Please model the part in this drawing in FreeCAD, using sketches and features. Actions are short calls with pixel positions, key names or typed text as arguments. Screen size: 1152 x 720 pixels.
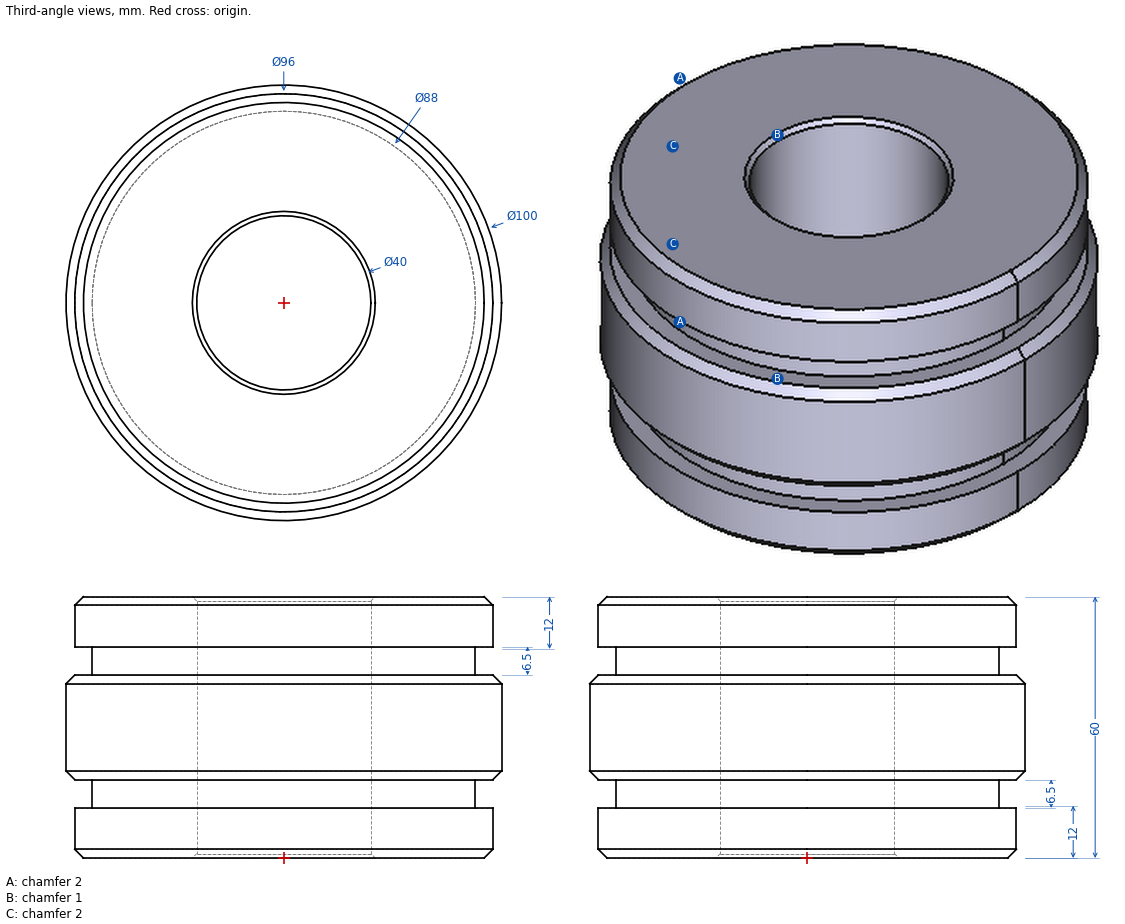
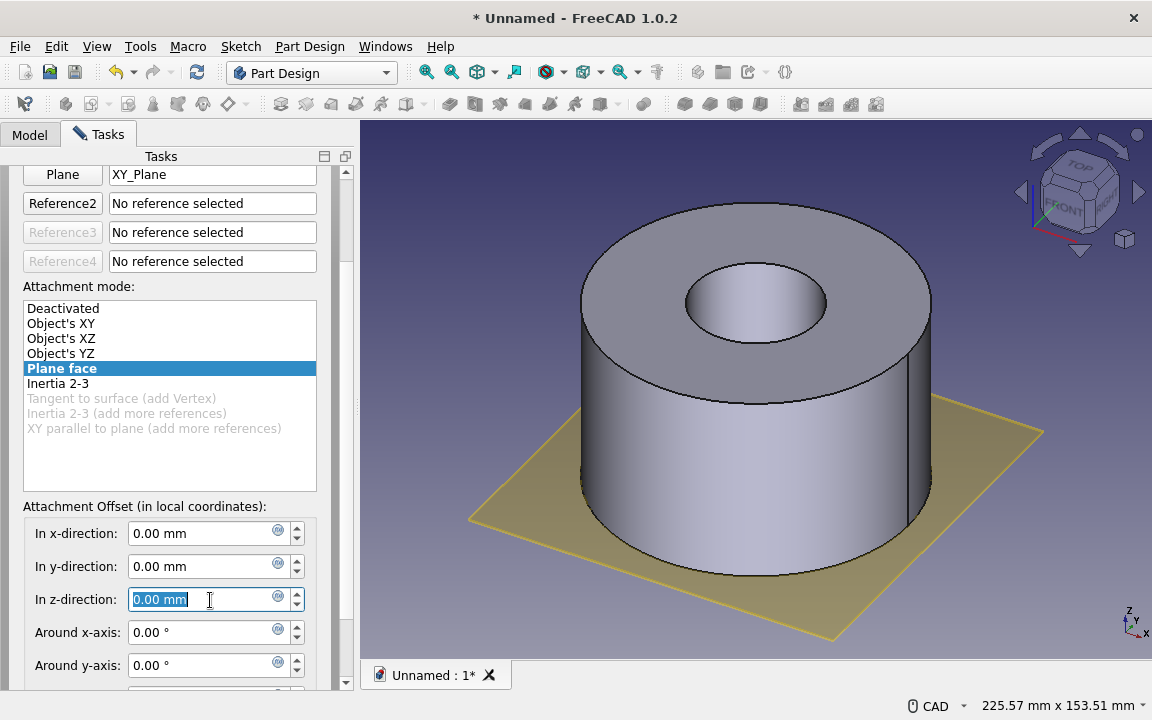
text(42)
key(Tab)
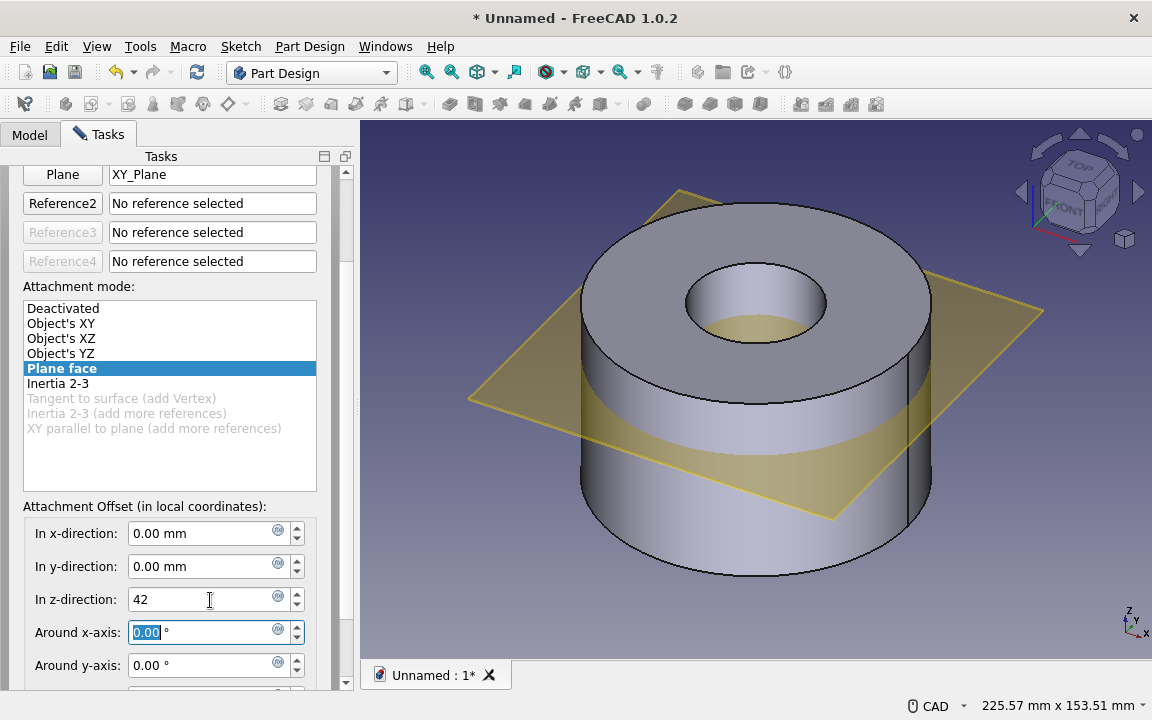
scroll(346, 428, up, 3)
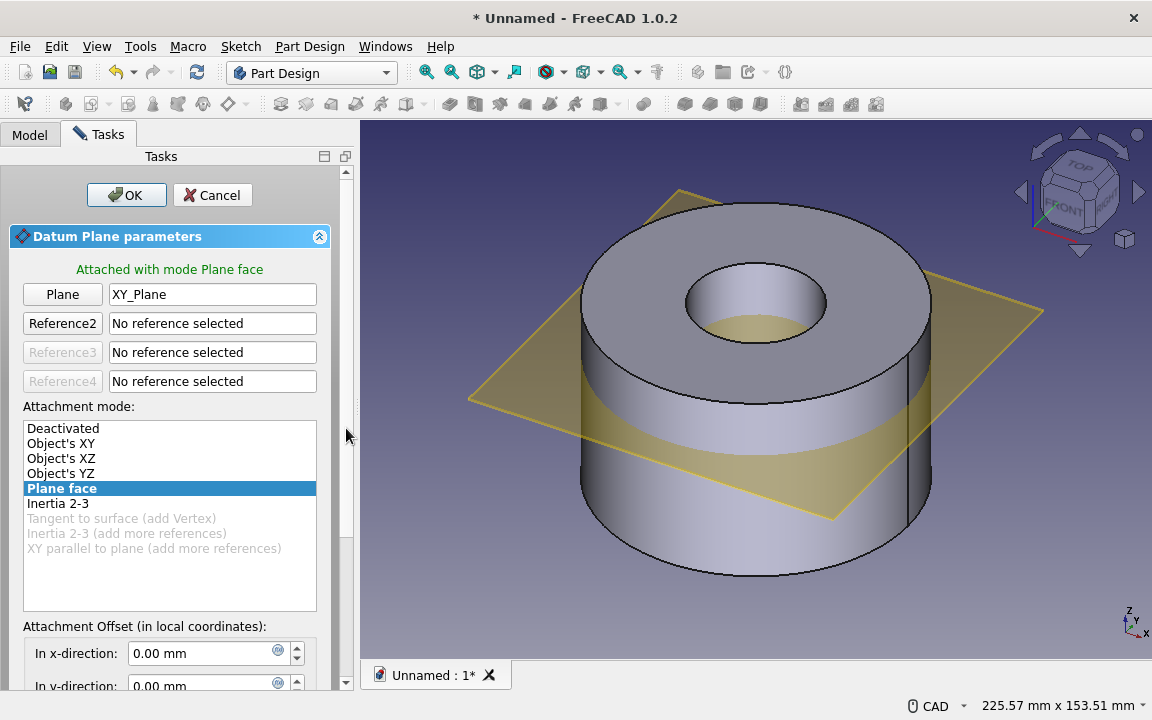
click(127, 195)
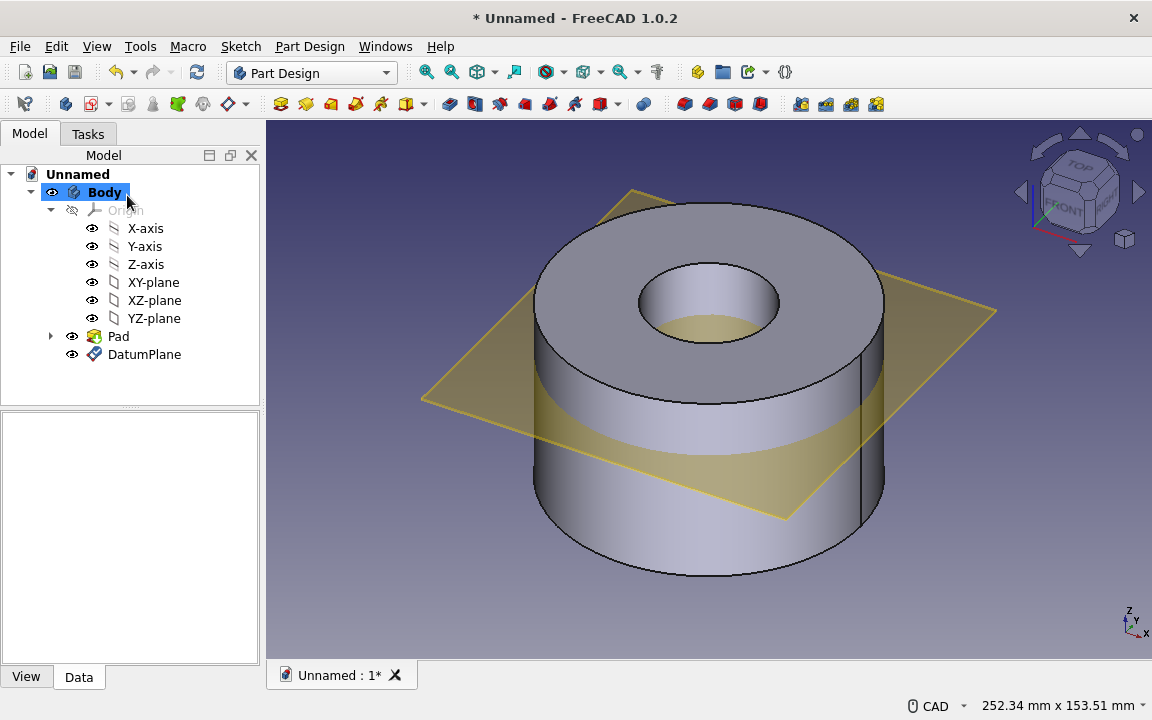
click(117, 354)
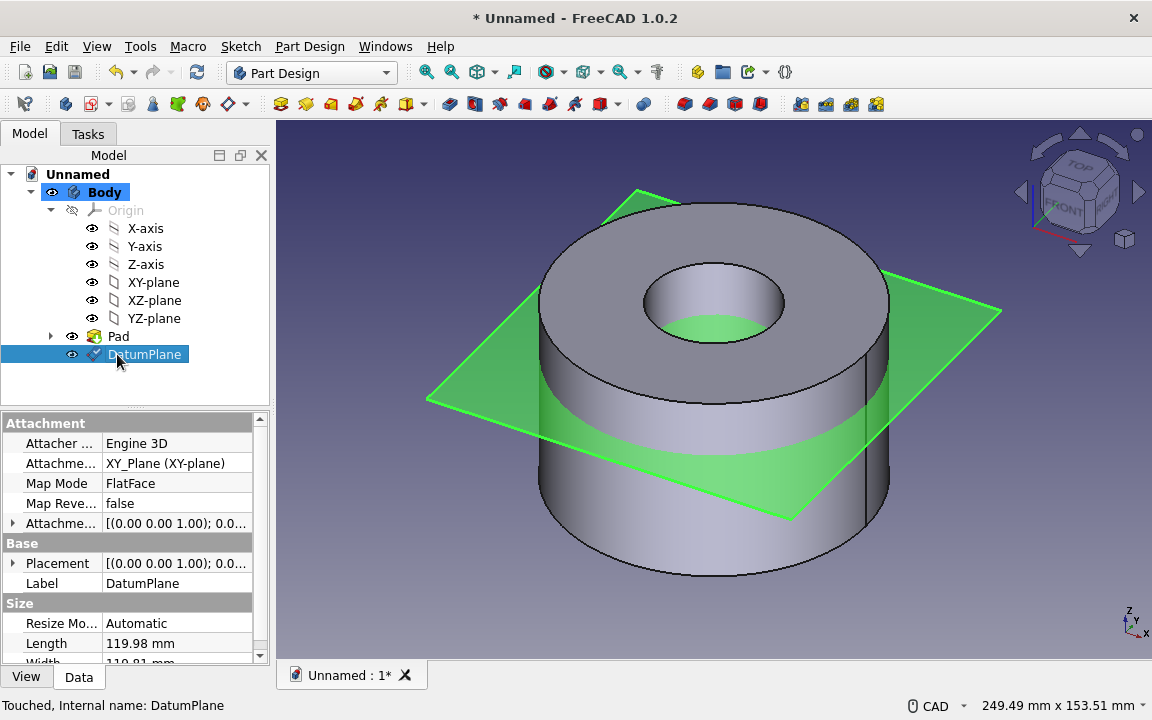
click(90, 104)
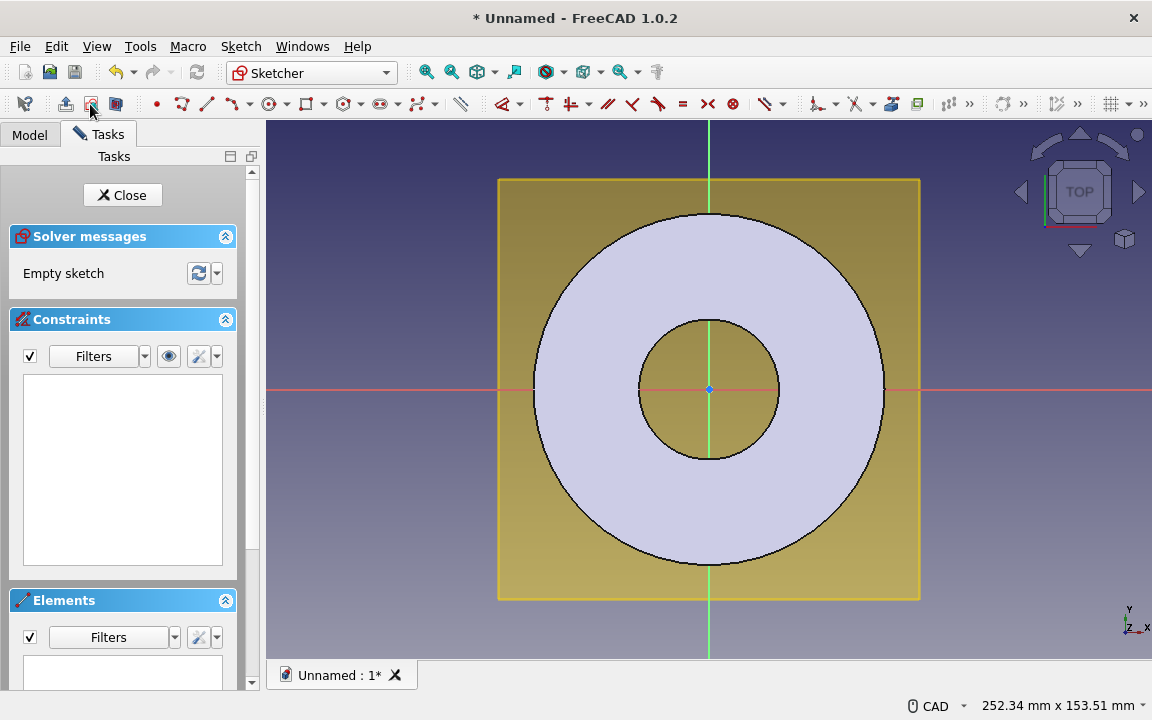
click(116, 104)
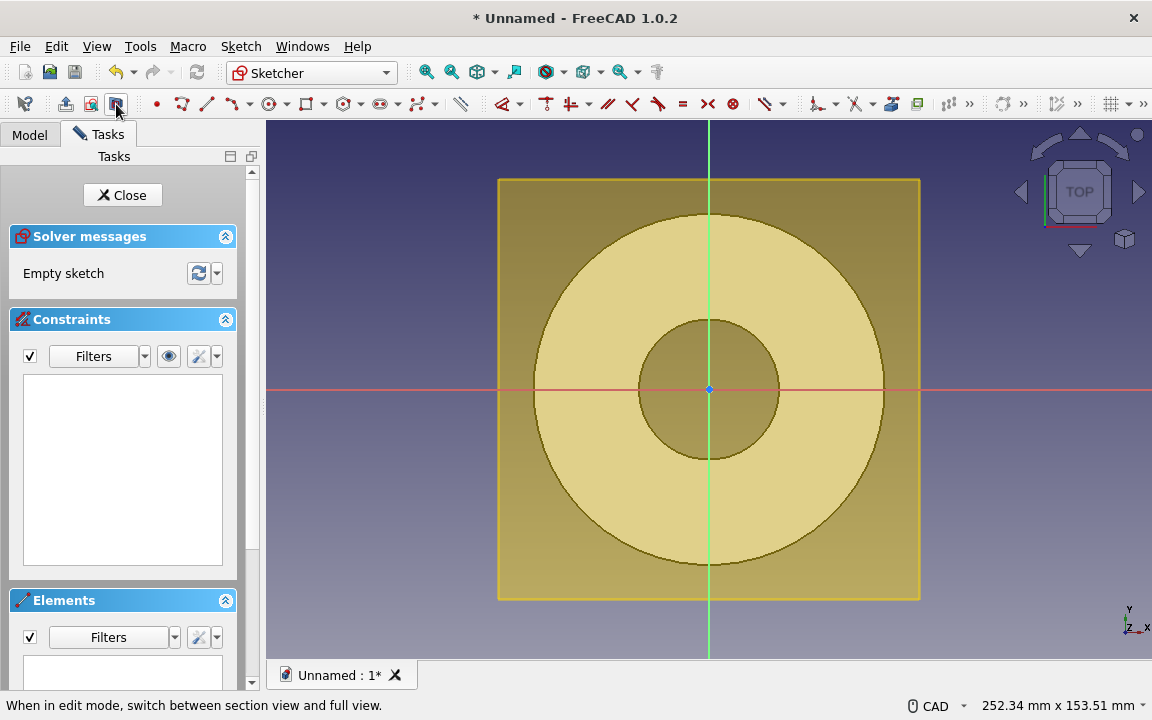
click(268, 104)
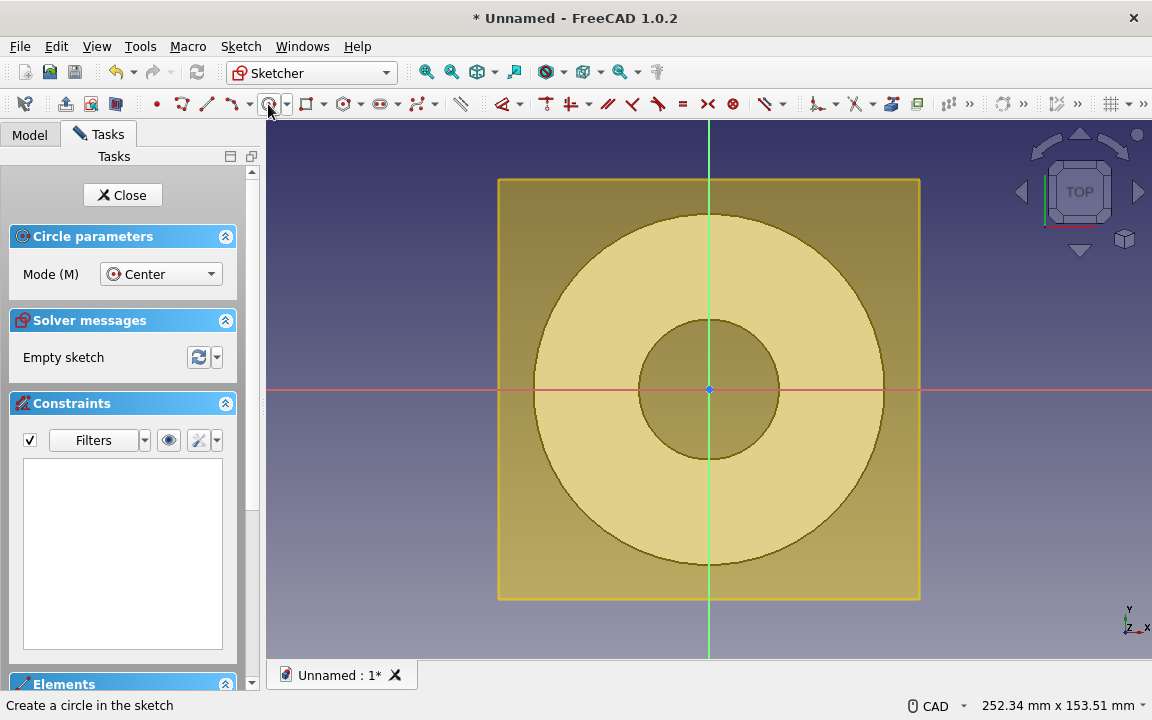
click(709, 390)
click(833, 265)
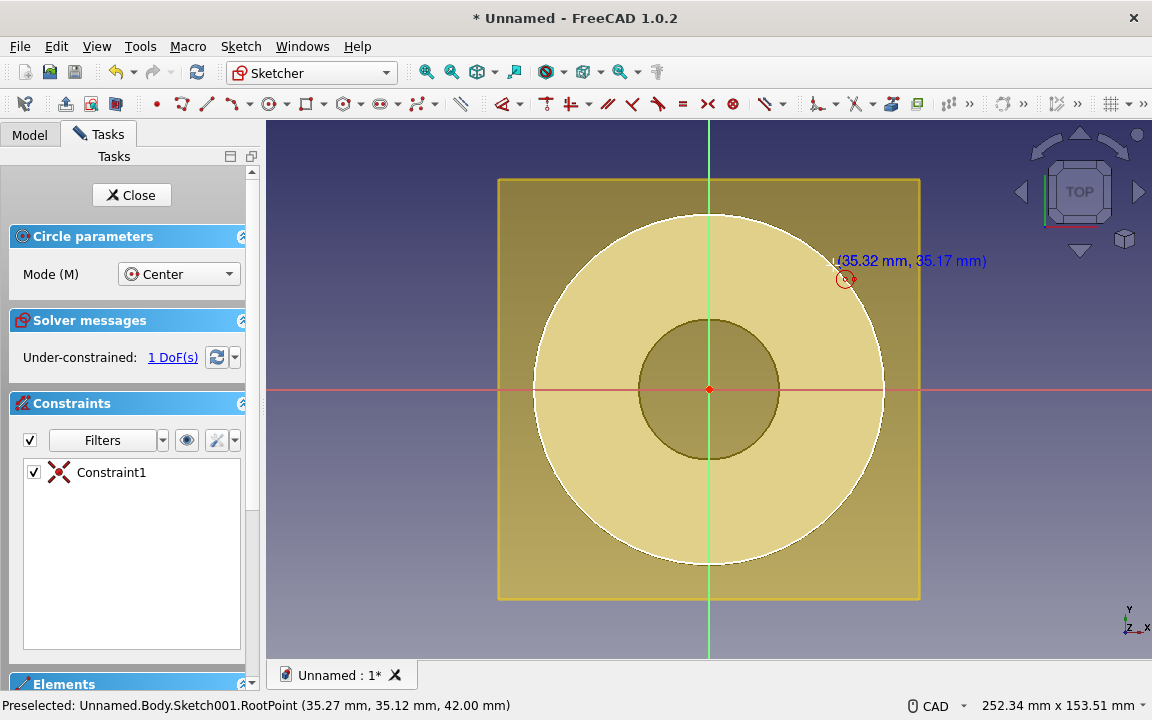
click(709, 390)
click(818, 280)
key(Escape)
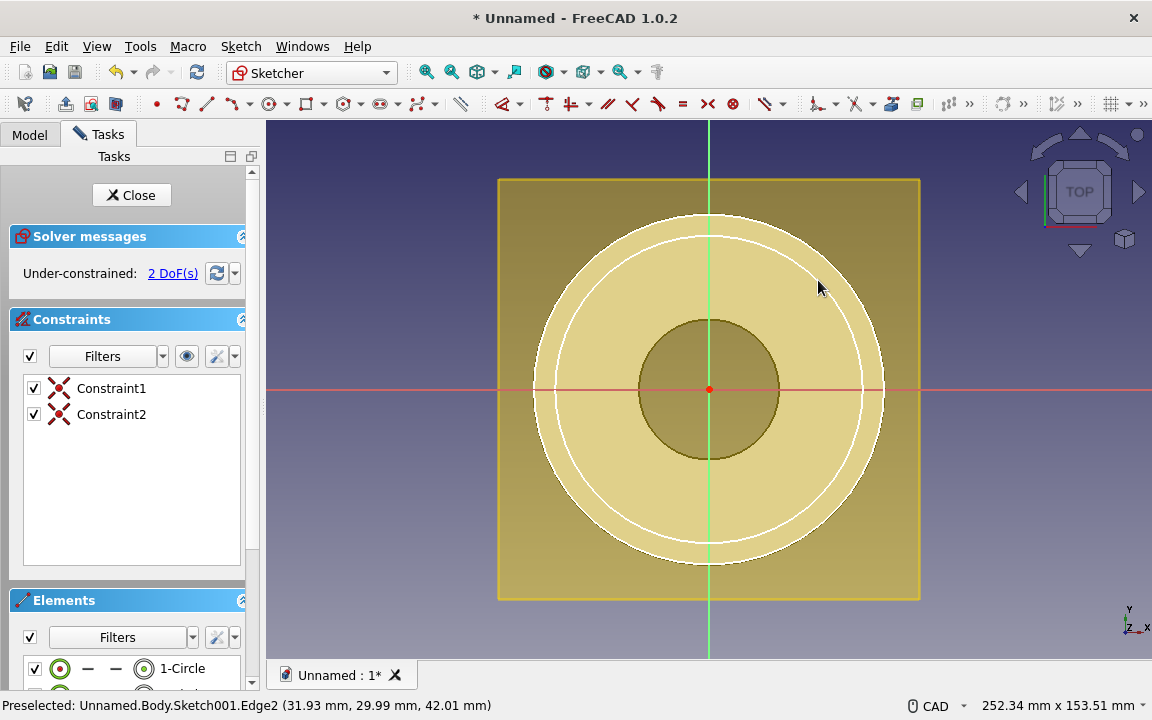
click(502, 104)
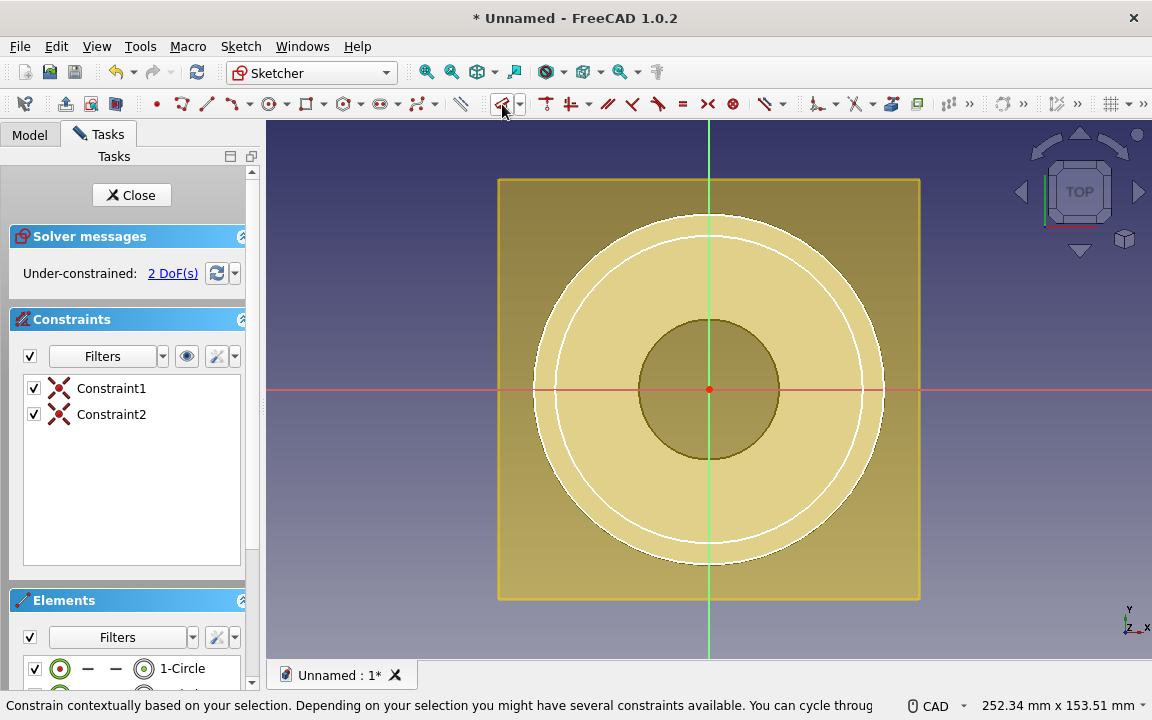
click(832, 265)
click(854, 242)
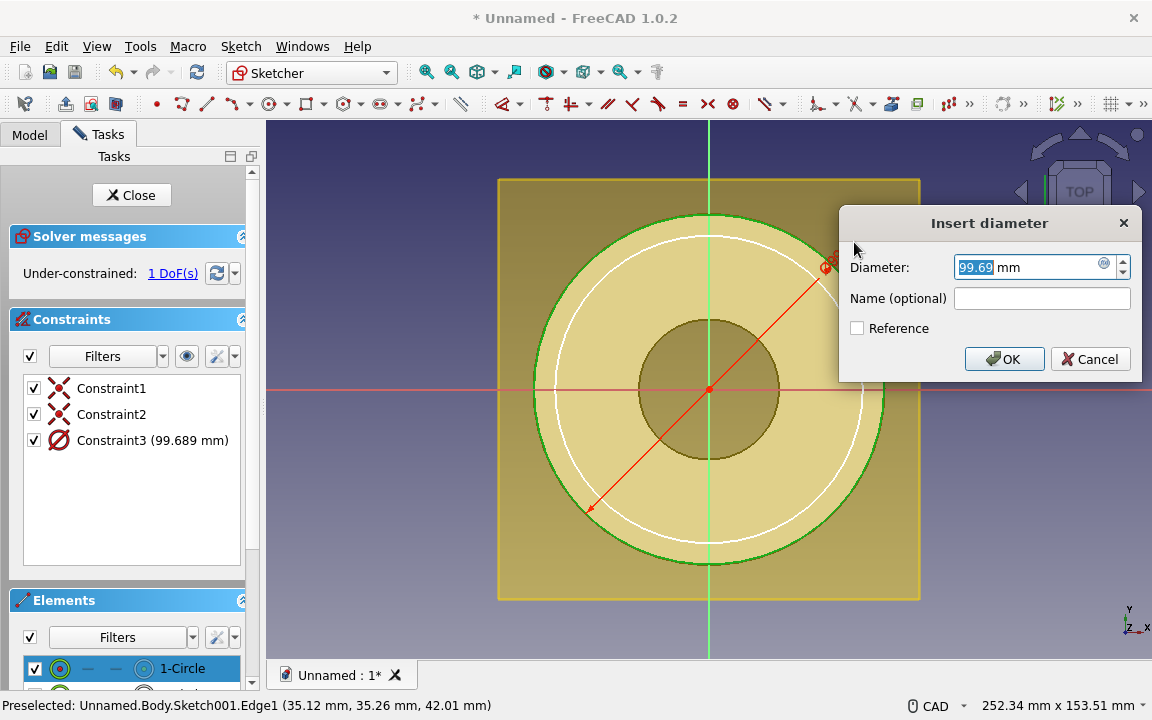
text(100)
key(Return)